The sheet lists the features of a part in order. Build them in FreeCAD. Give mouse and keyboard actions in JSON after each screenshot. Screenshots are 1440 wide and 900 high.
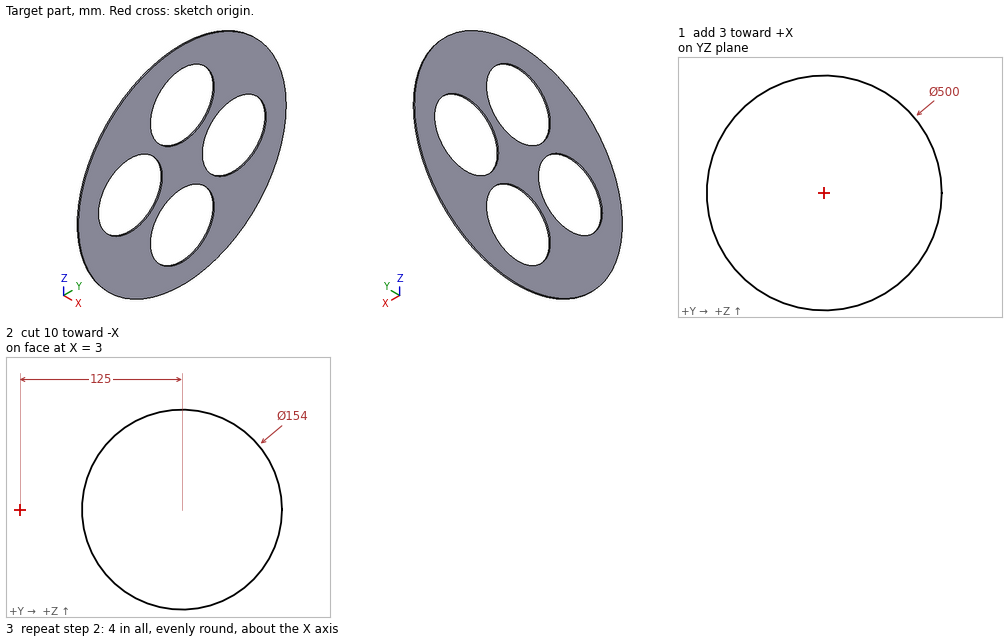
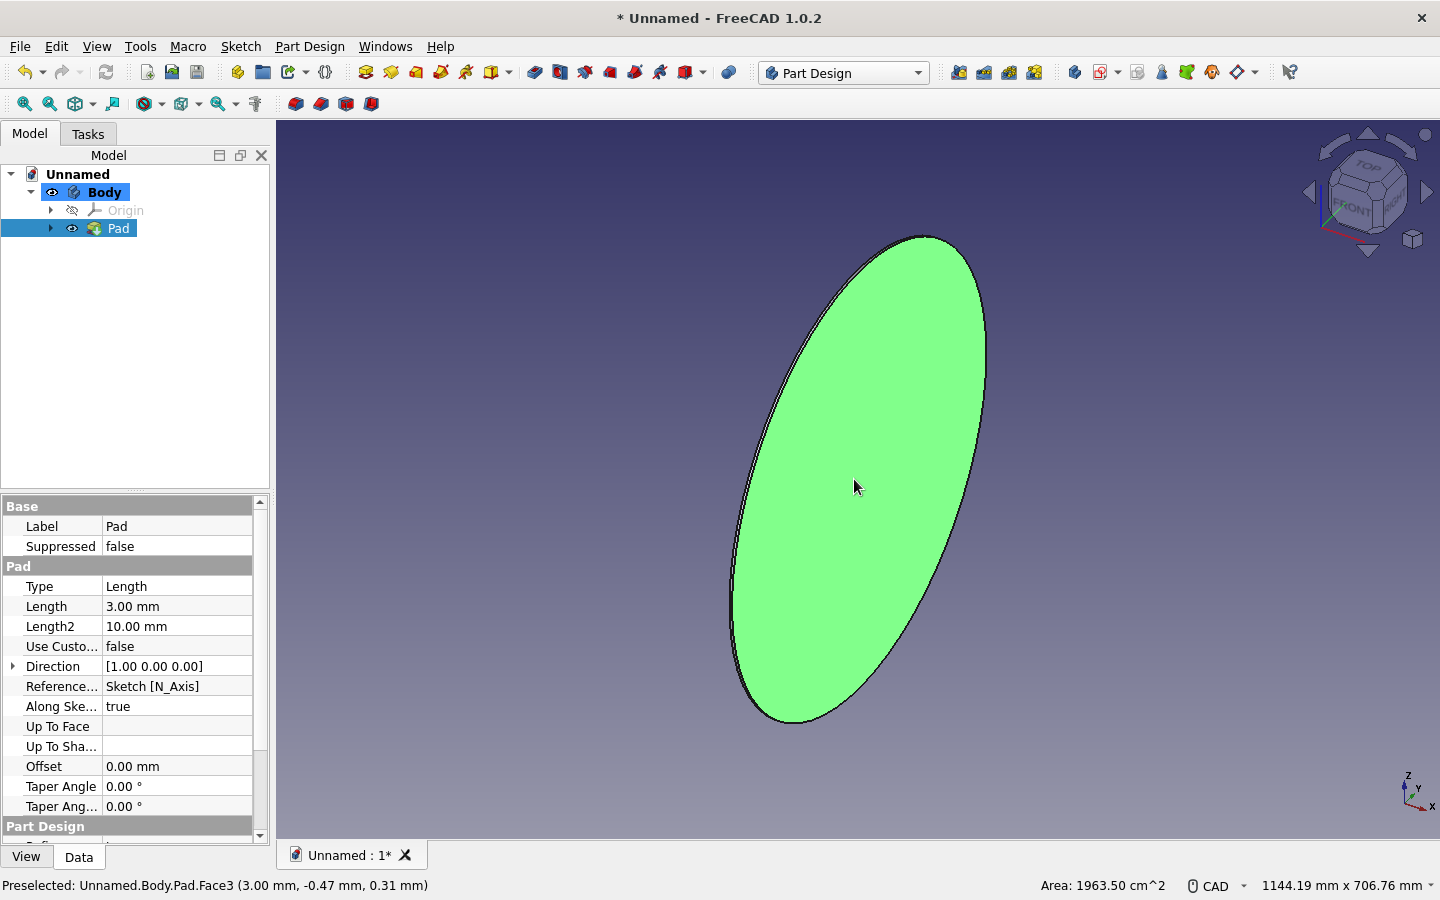
{"action": "left_click", "coordinate": [1100, 72]}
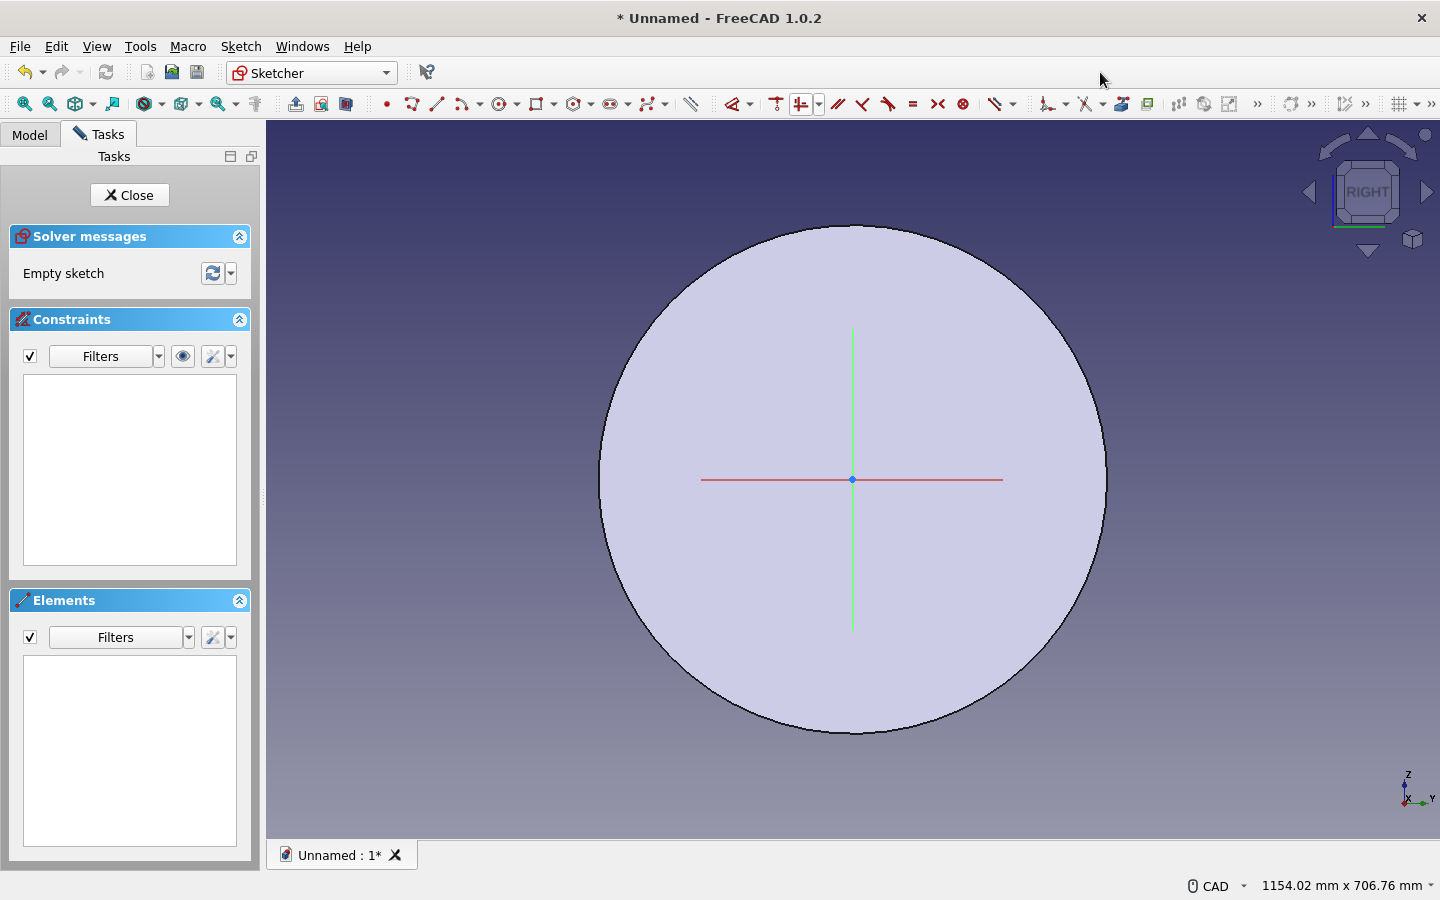
{"action": "scroll", "coordinate": [1055, 480], "scroll_direction": "up", "scroll_amount": 5}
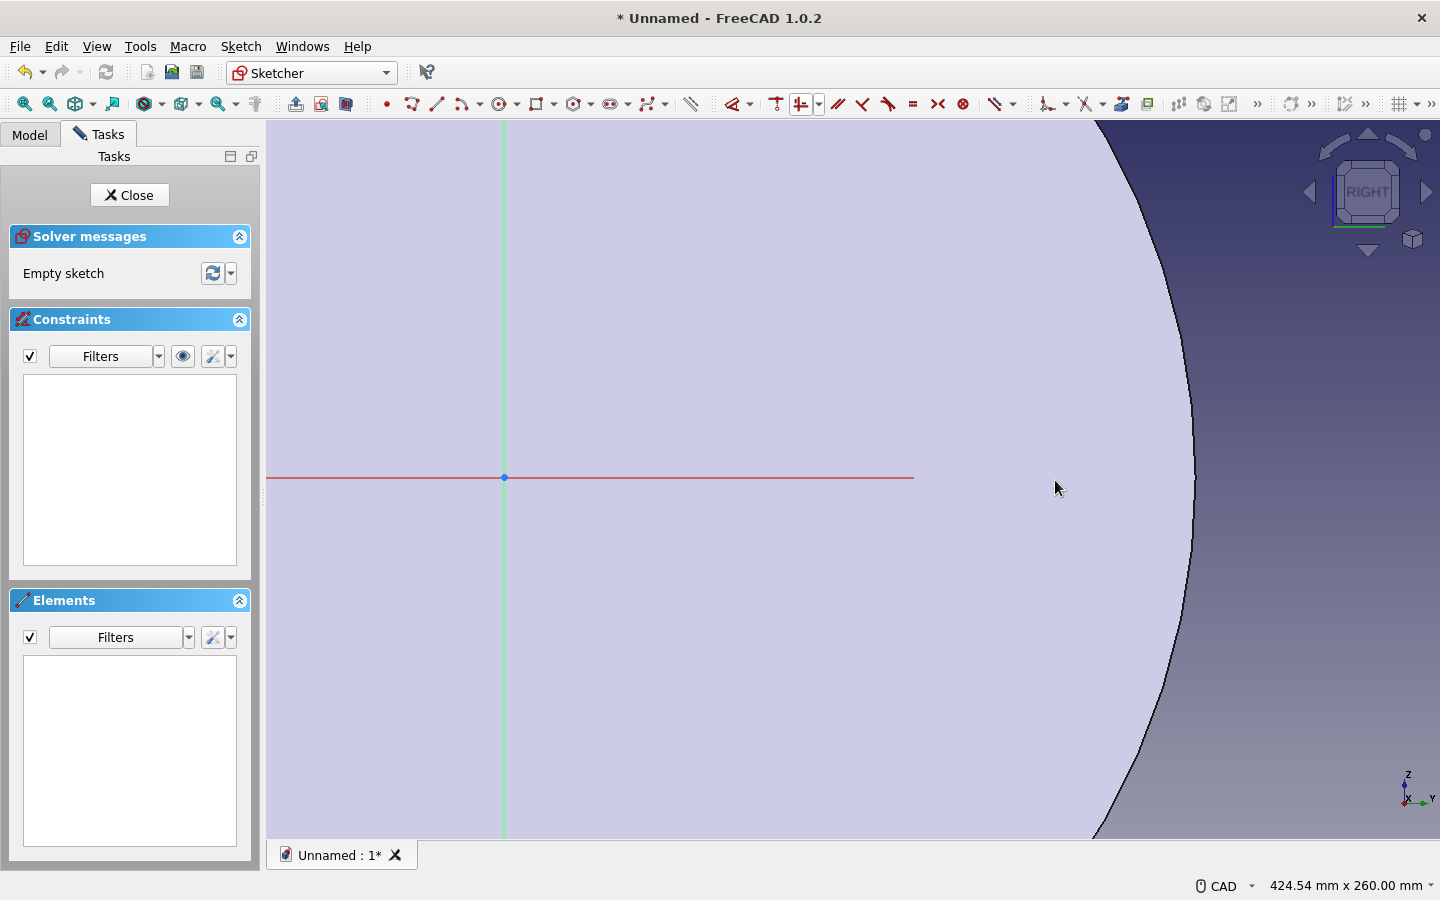
{"action": "left_click", "coordinate": [498, 104]}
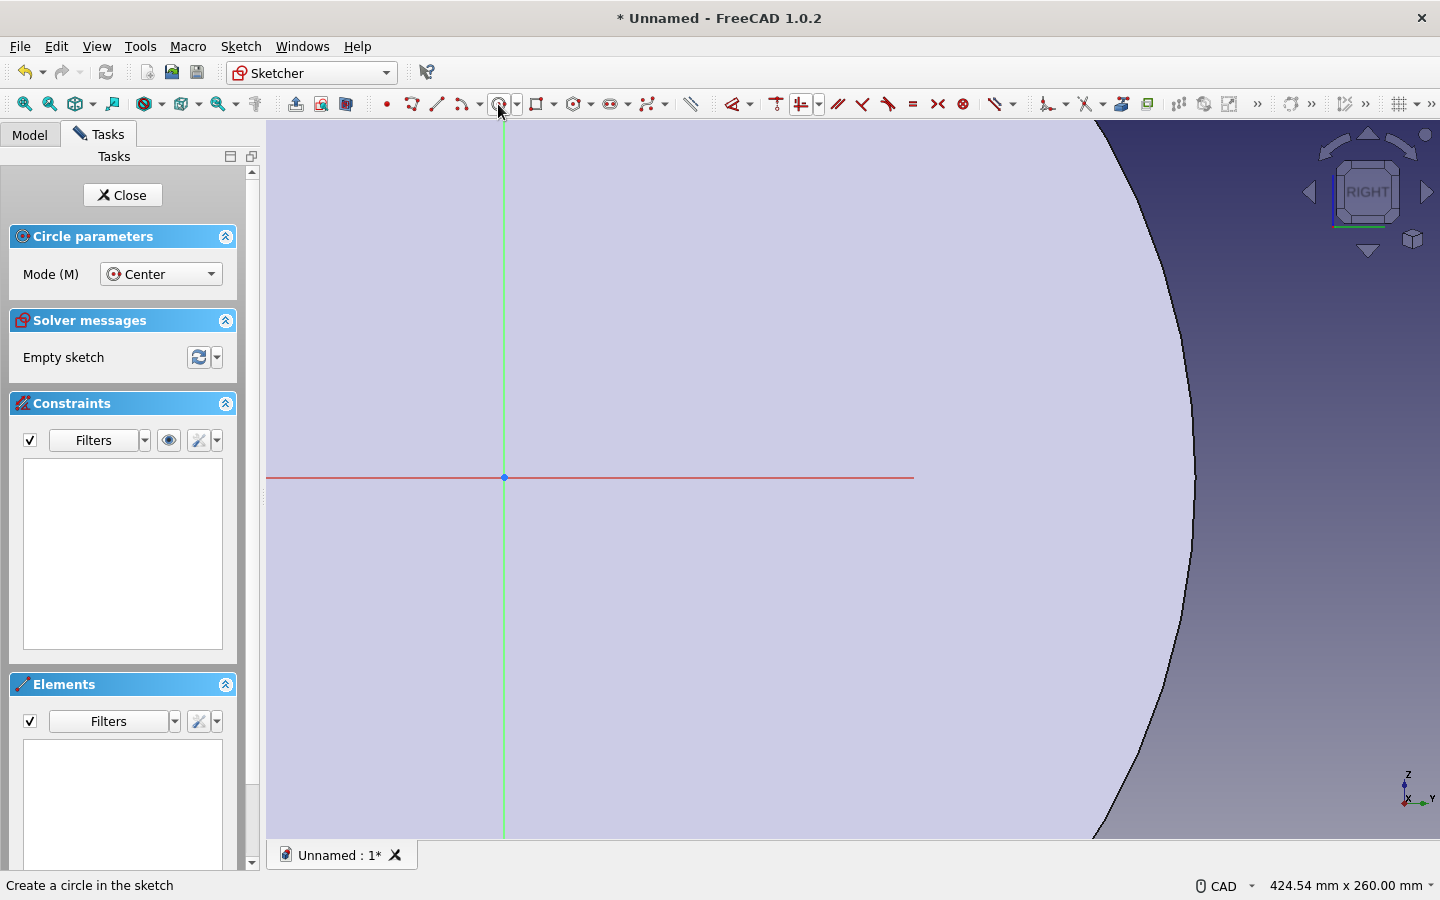
{"action": "left_click", "coordinate": [850, 478]}
{"action": "left_click", "coordinate": [1001, 327]}
{"action": "key", "text": "Escape"}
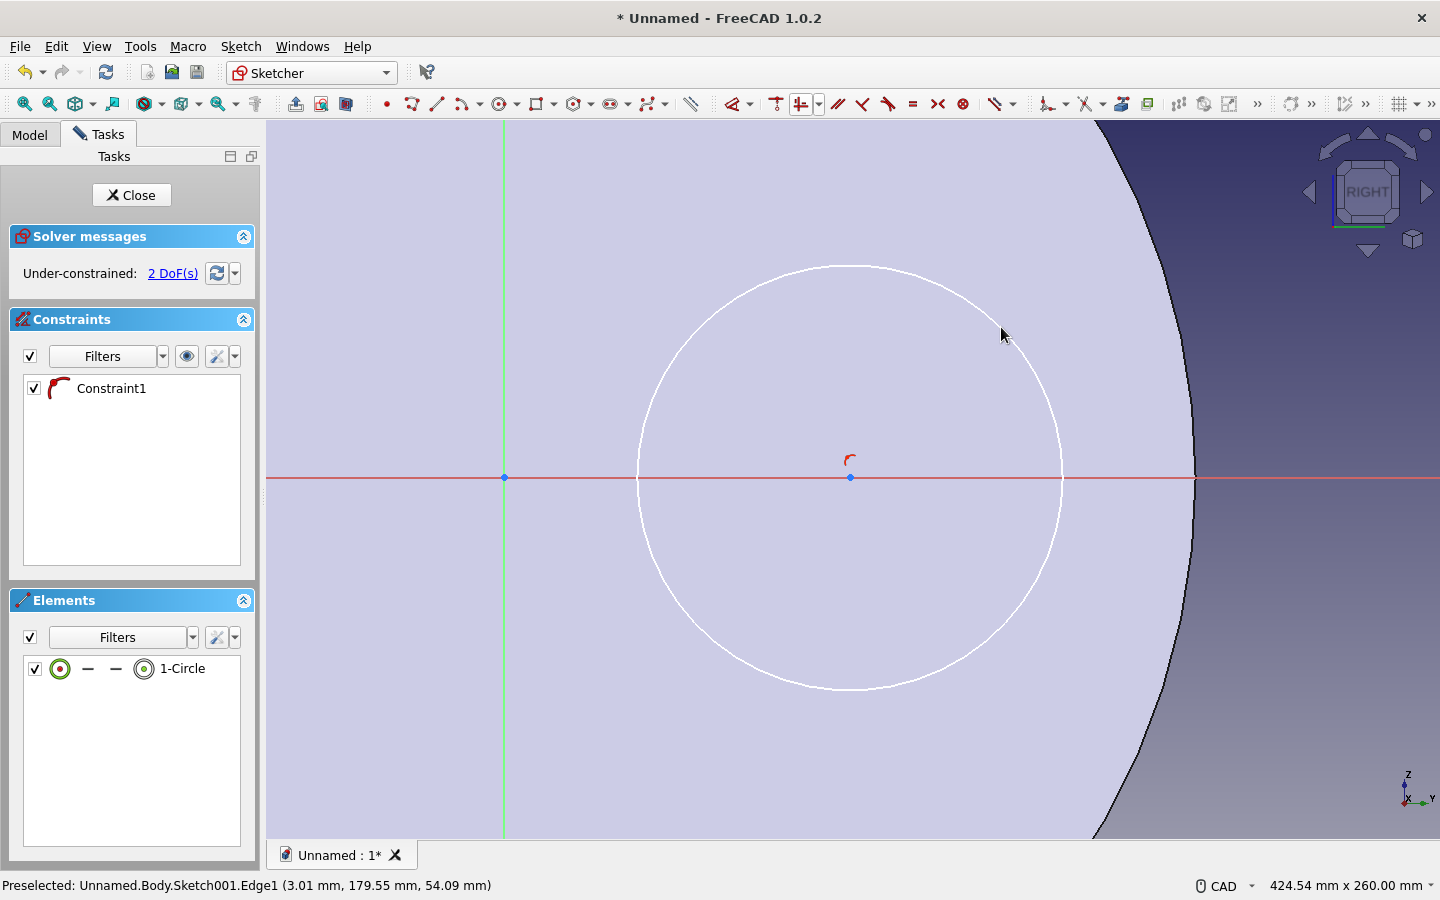
{"action": "left_click", "coordinate": [732, 104]}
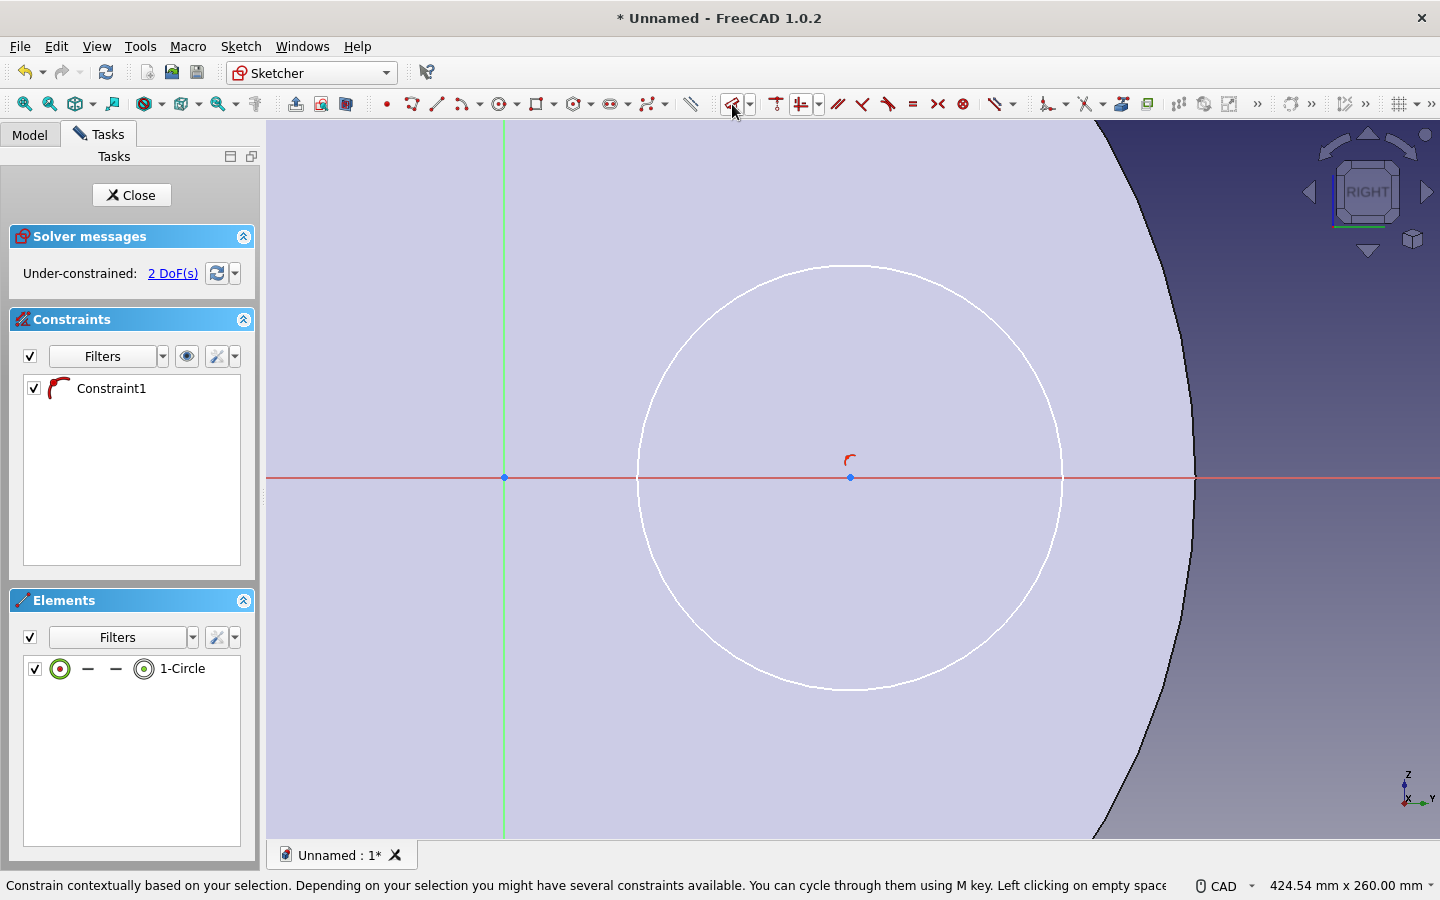
{"action": "left_click", "coordinate": [1000, 327]}
{"action": "left_click", "coordinate": [1023, 304]}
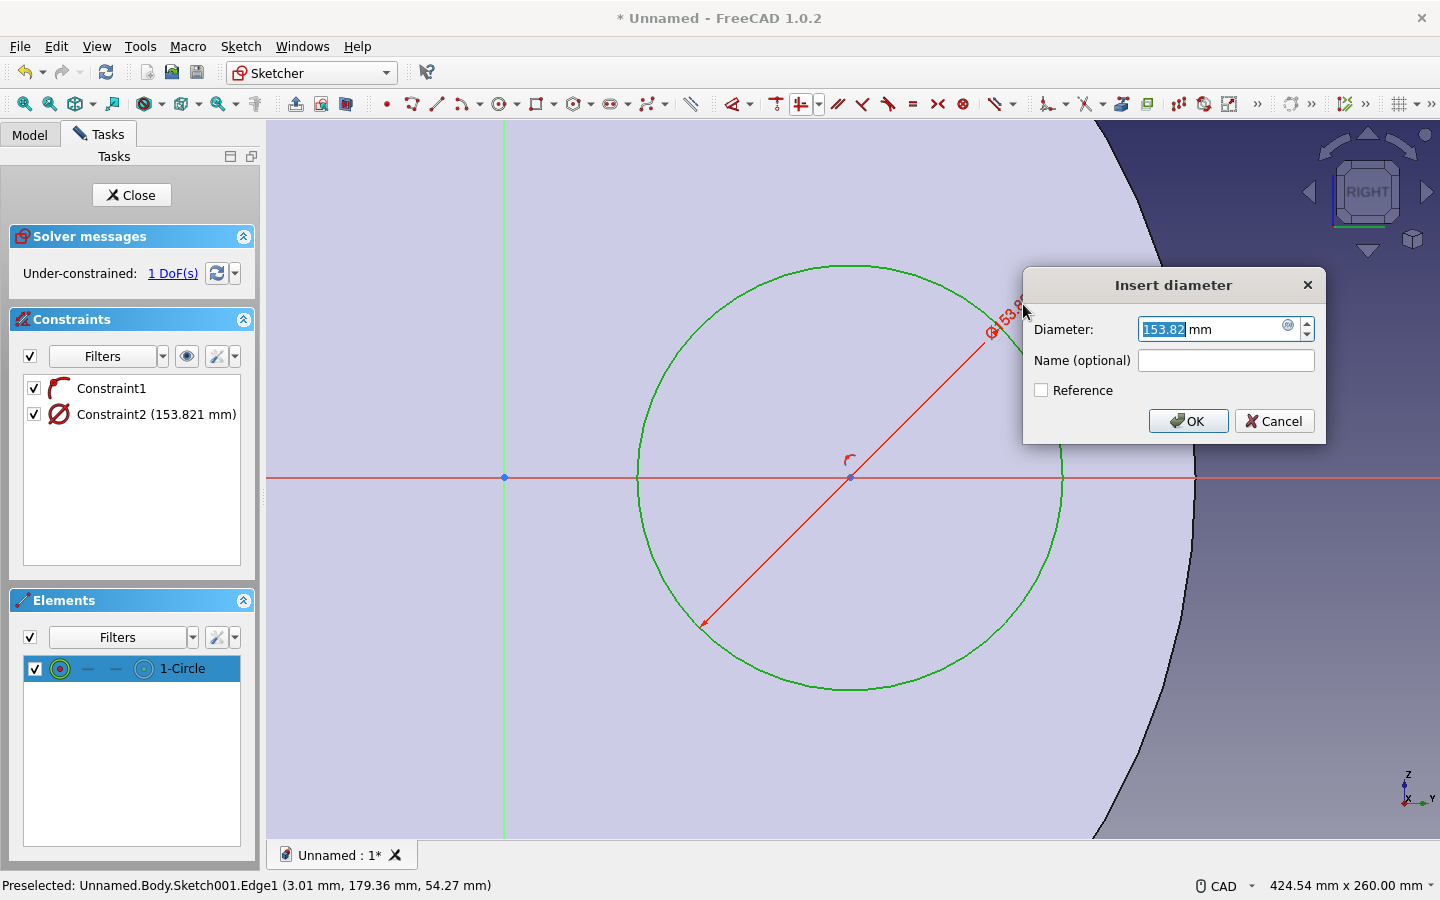
{"action": "type", "text": "154"}
{"action": "key", "text": "Return"}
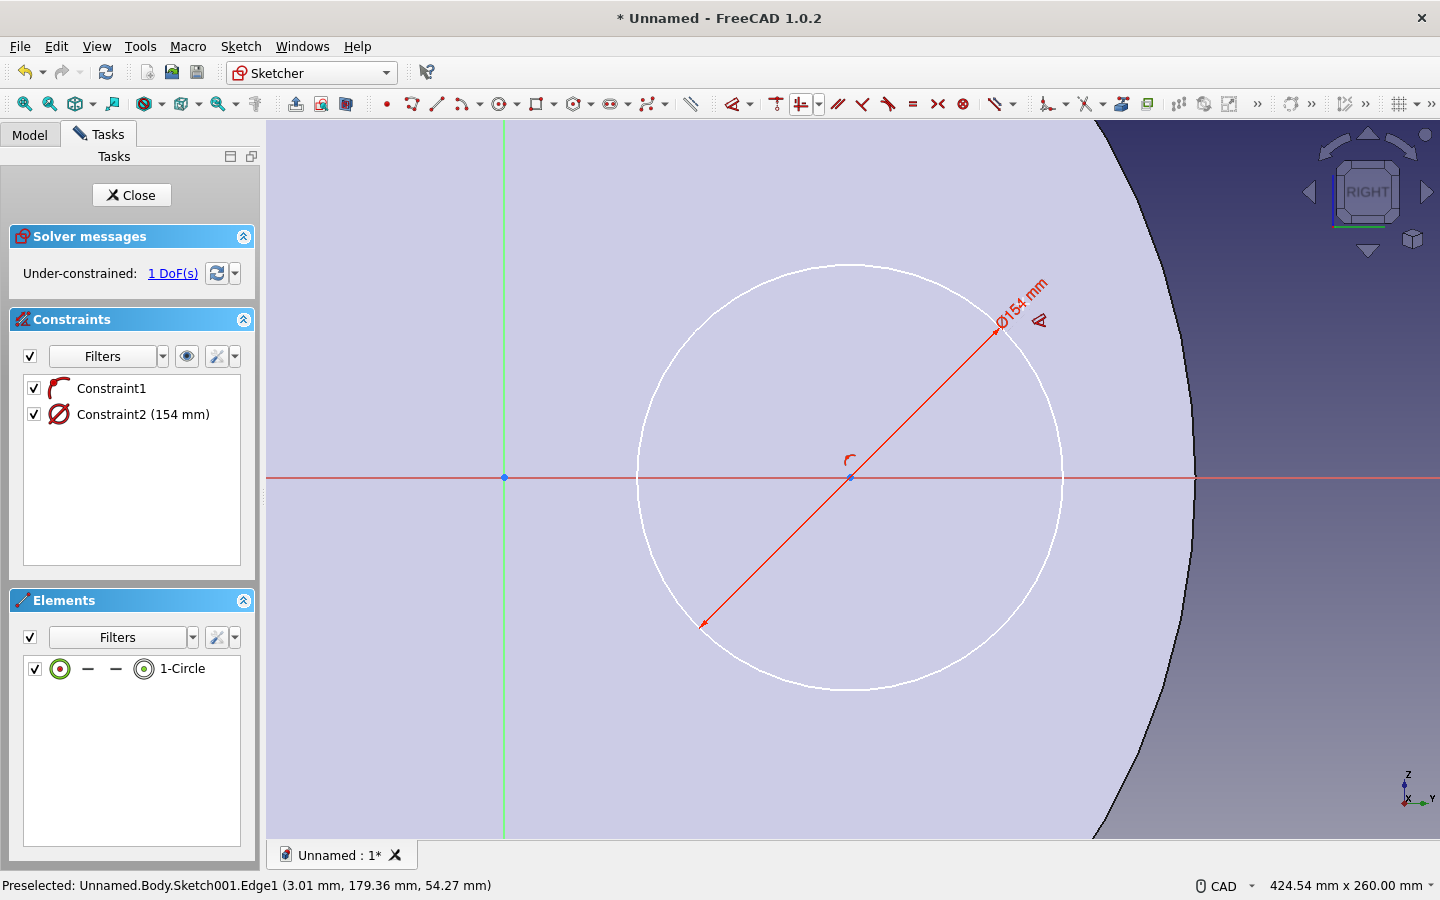
{"action": "left_click", "coordinate": [850, 478]}
{"action": "left_click", "coordinate": [677, 512]}